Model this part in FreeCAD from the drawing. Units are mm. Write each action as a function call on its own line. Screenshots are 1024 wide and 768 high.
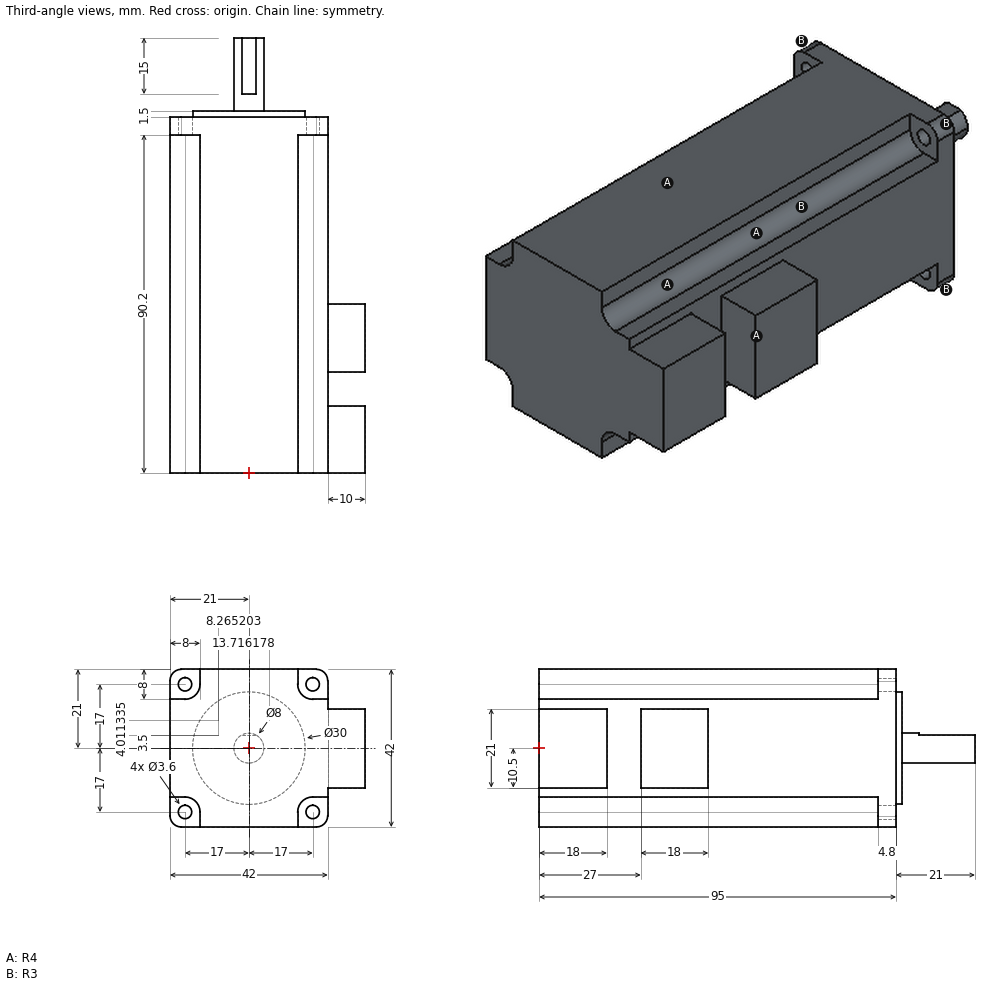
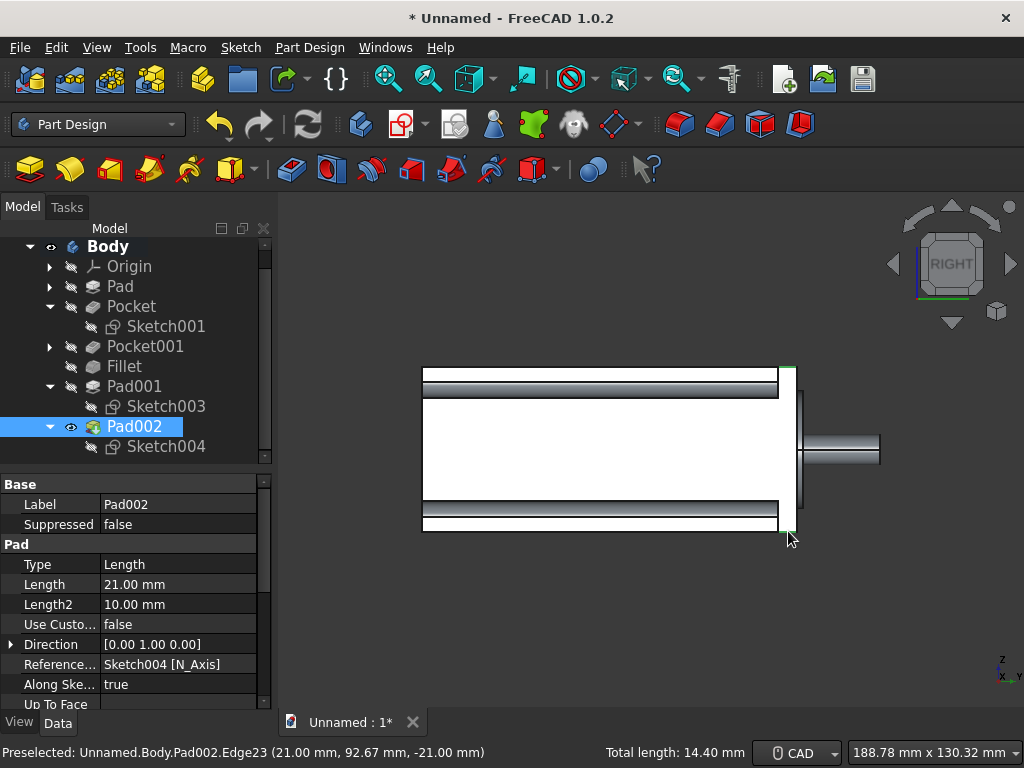
scroll(788, 531, up, 4)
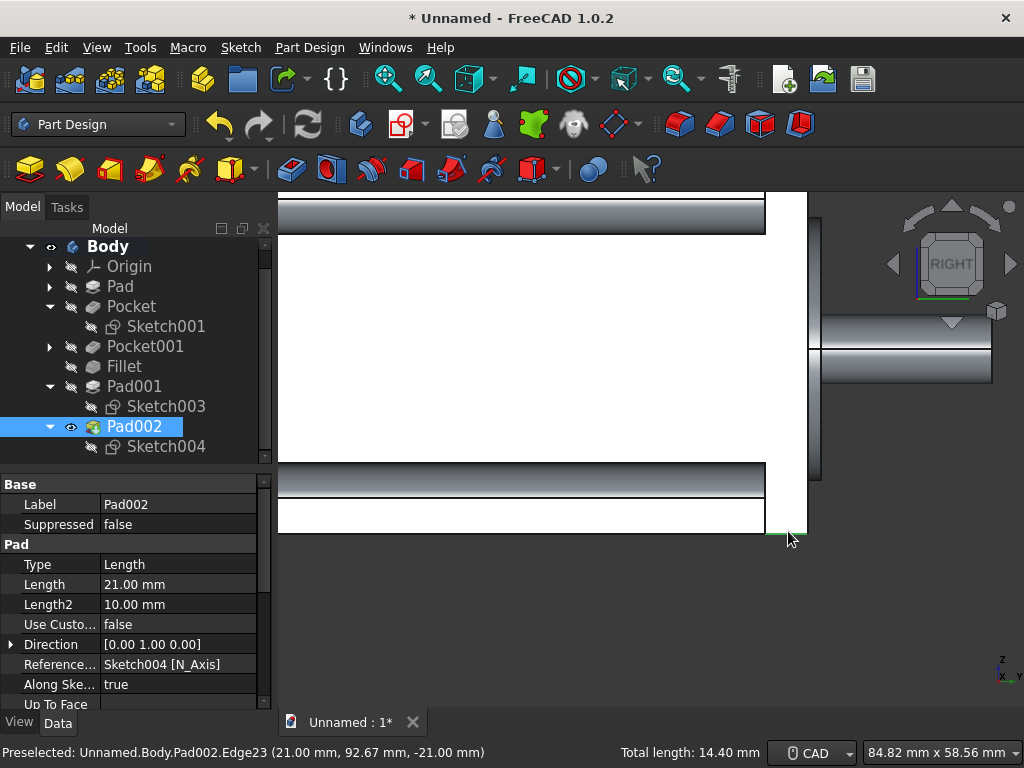
click(390, 80)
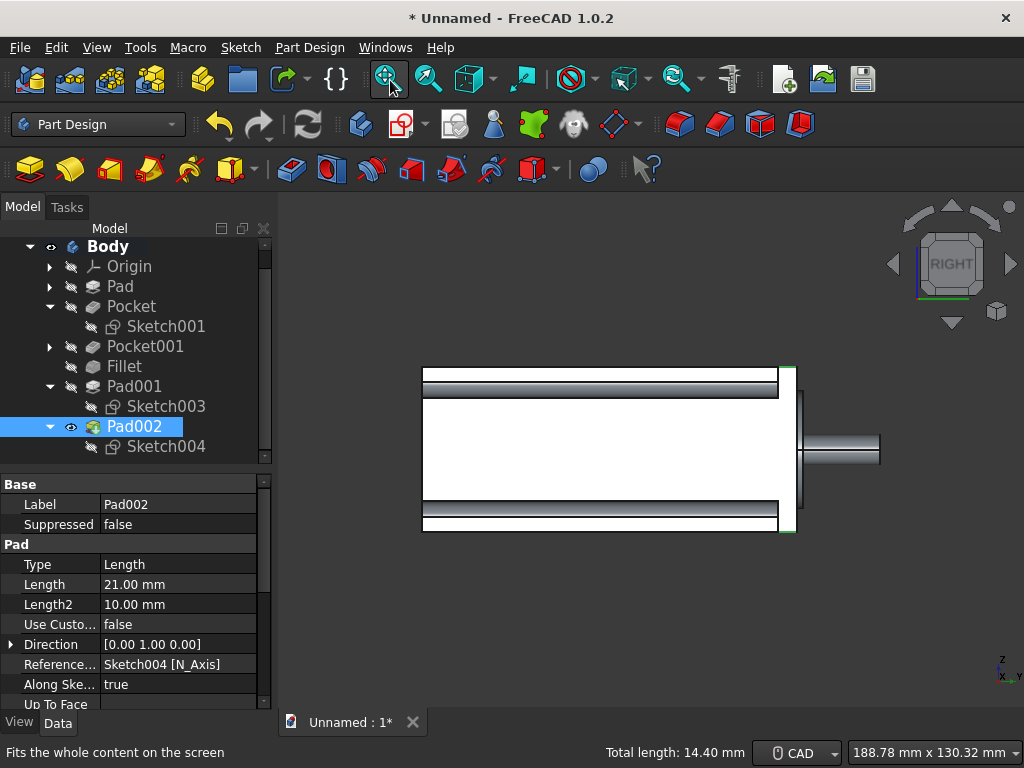
key(5)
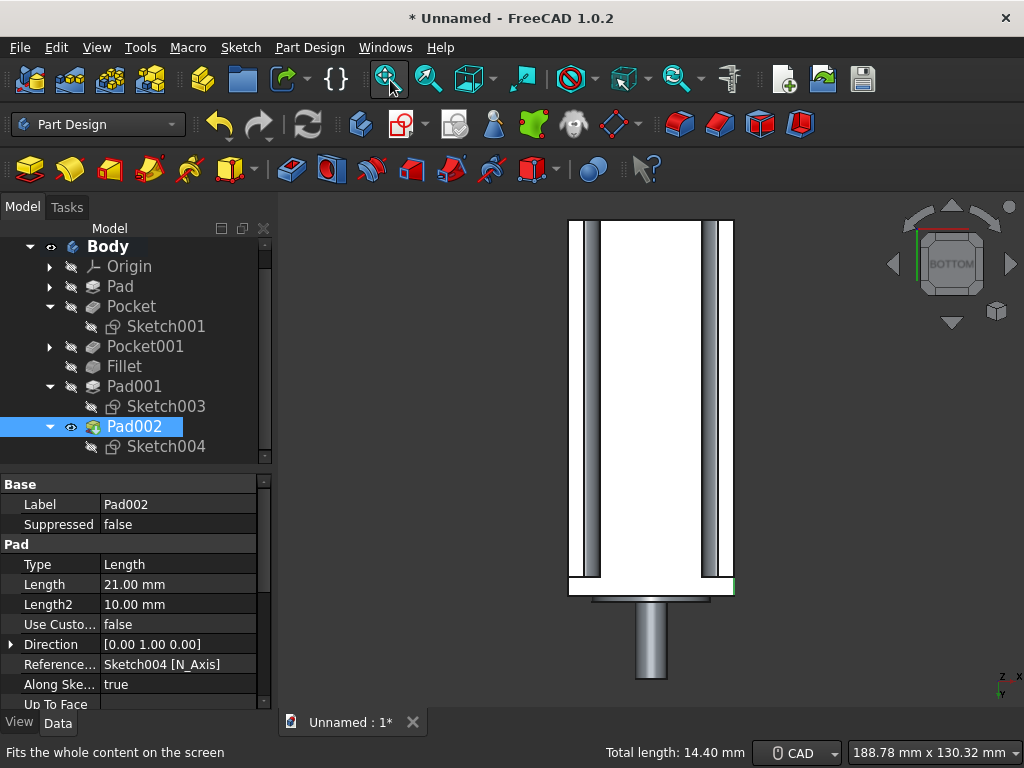
click(568, 585, ctrl)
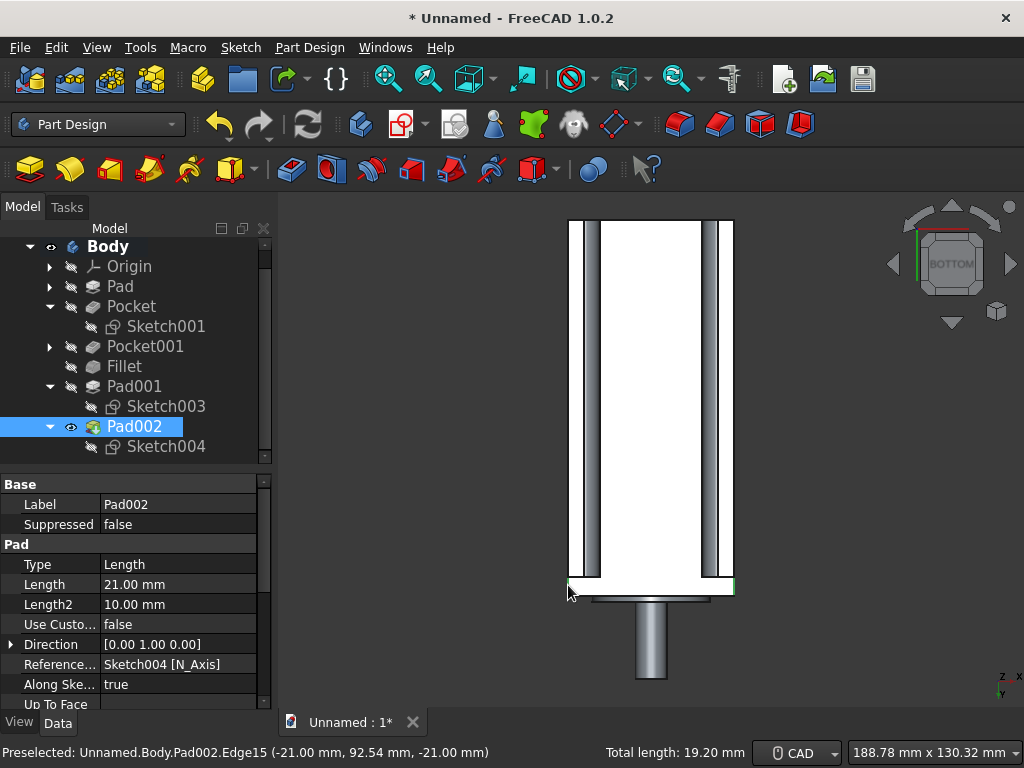
click(680, 124)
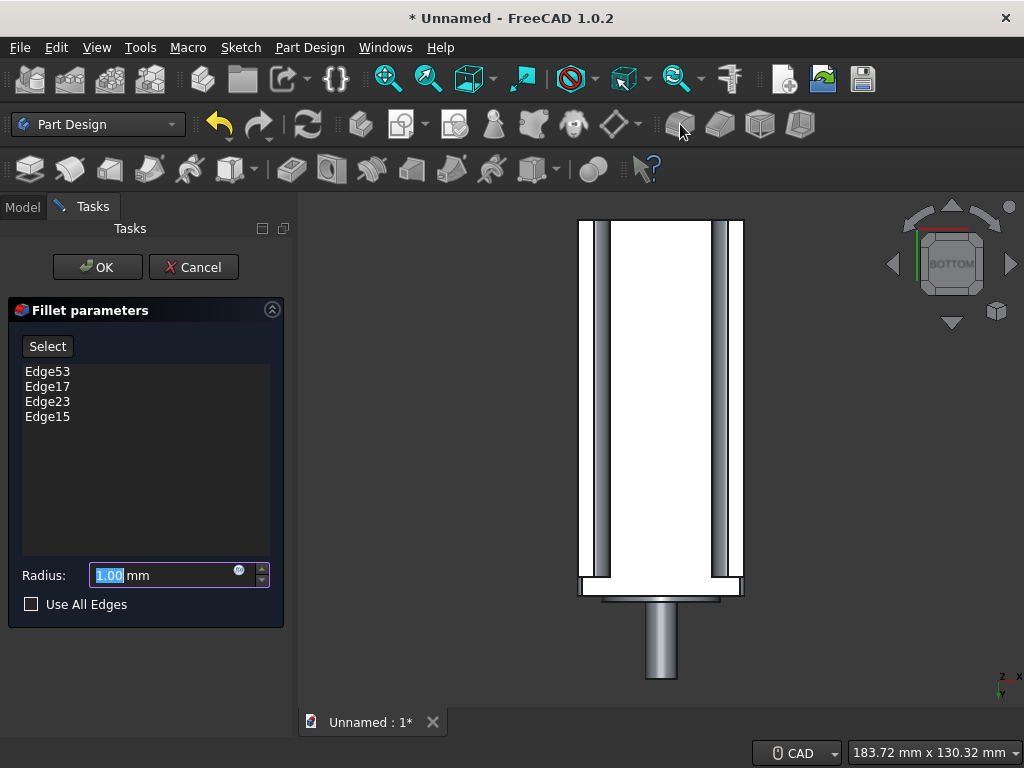
text(3)
key(Tab)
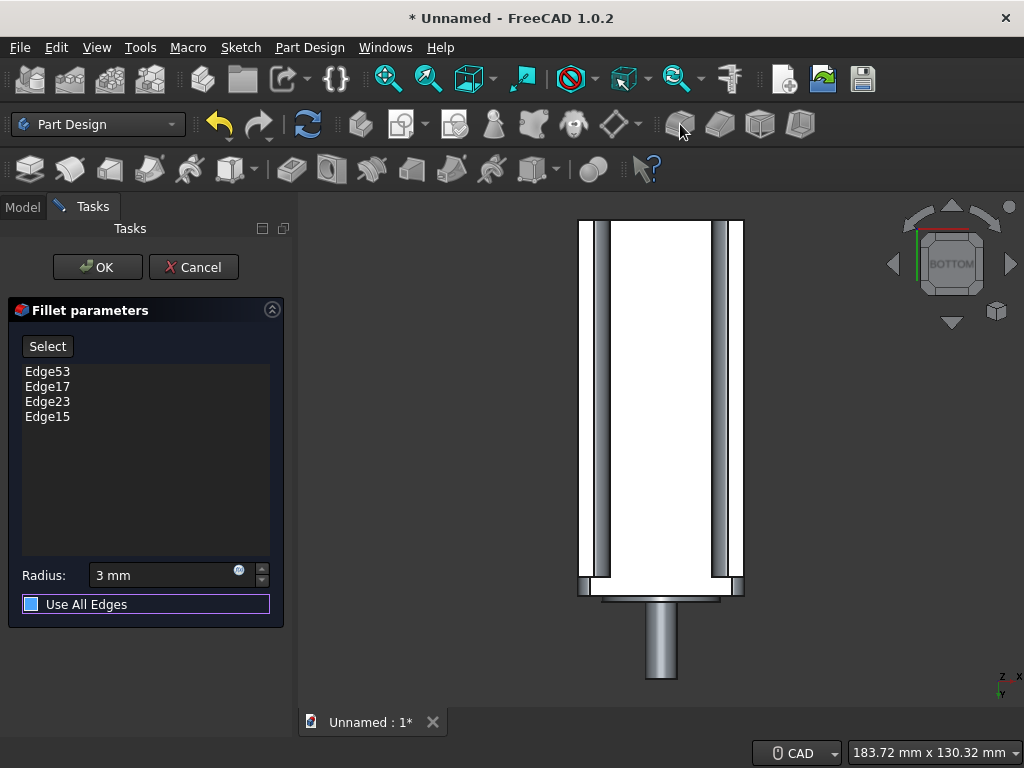
click(98, 267)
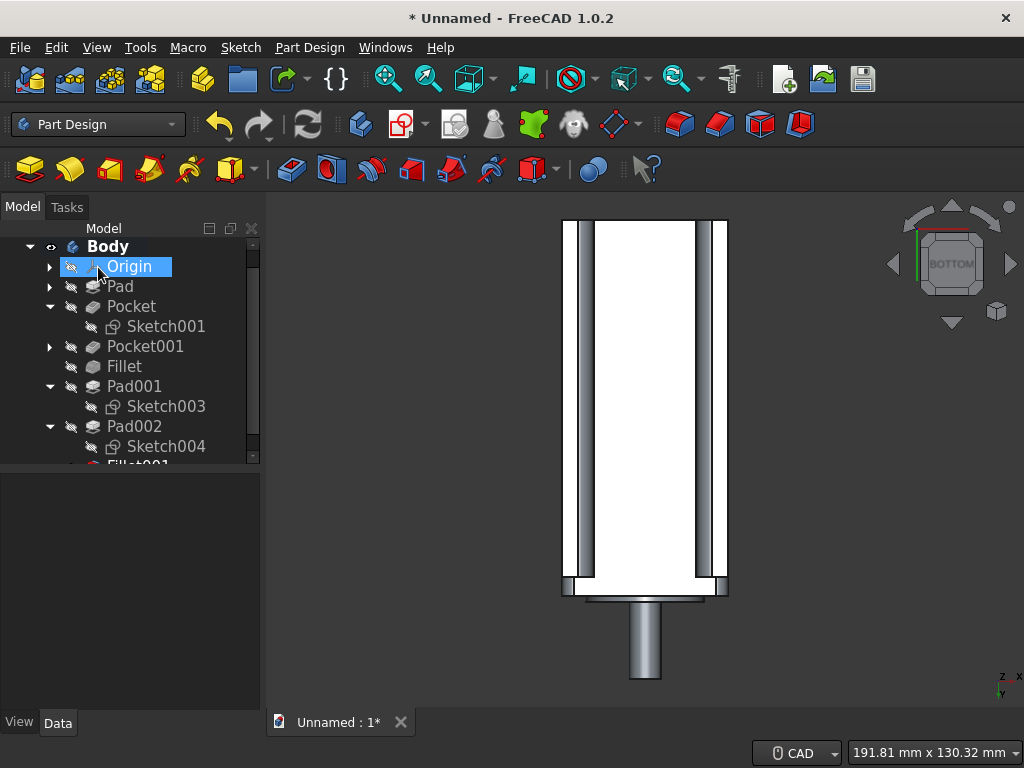
key(0)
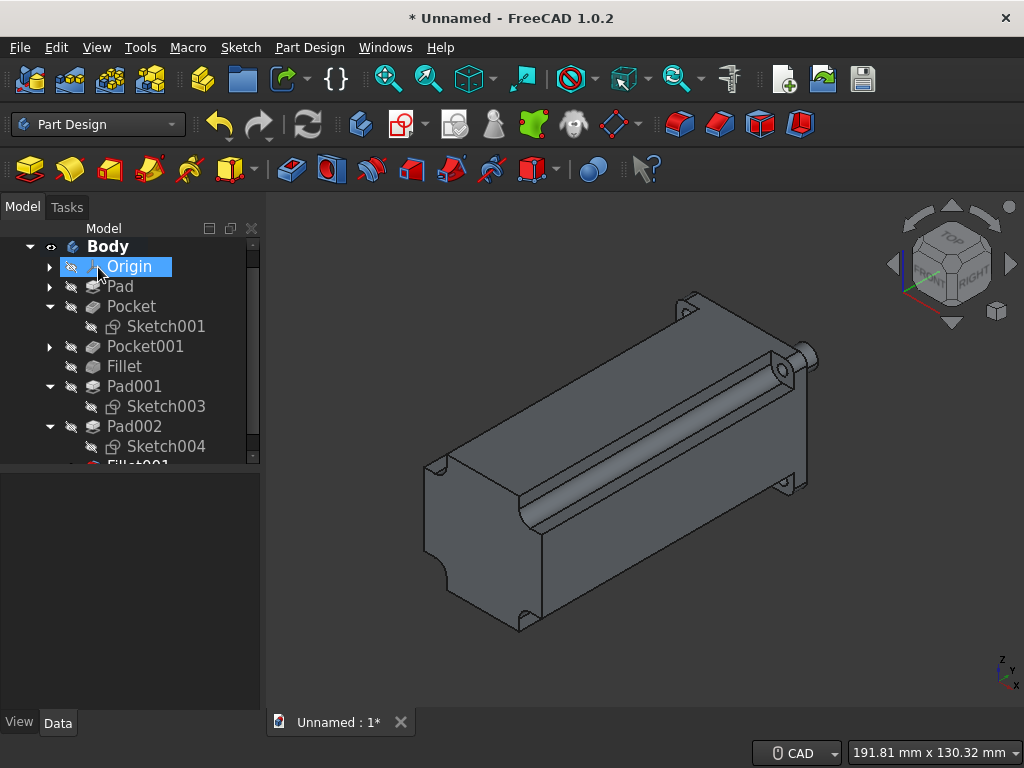
click(750, 456)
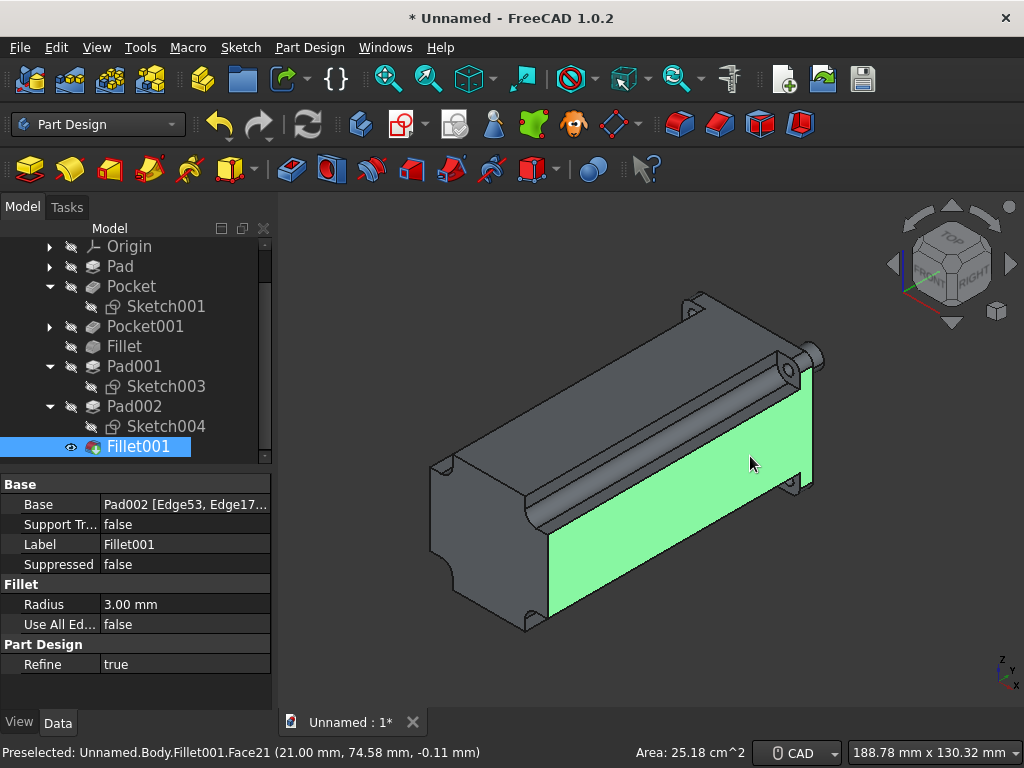
click(402, 124)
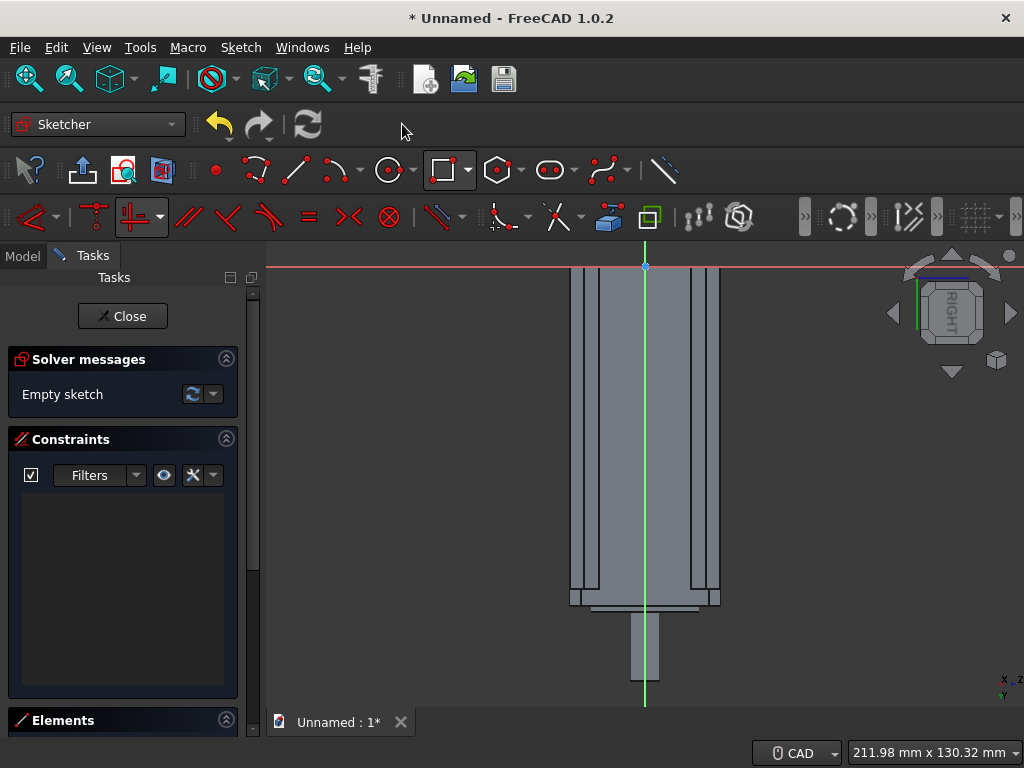
scroll(576, 474, down, 5)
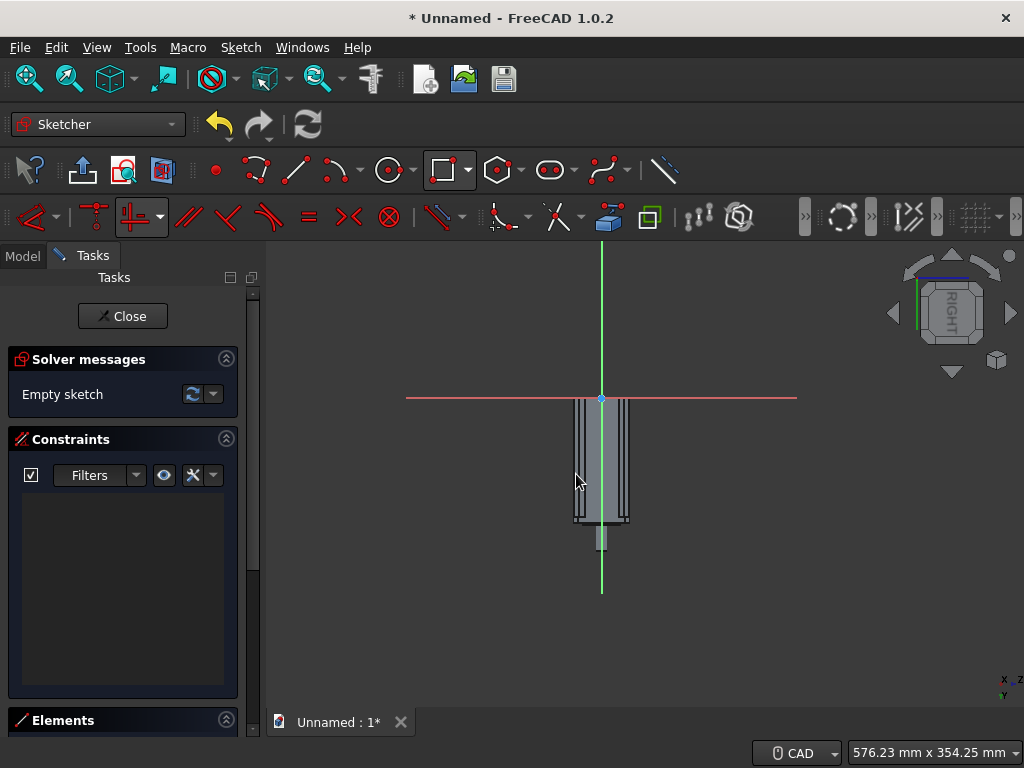
scroll(608, 416, up, 8)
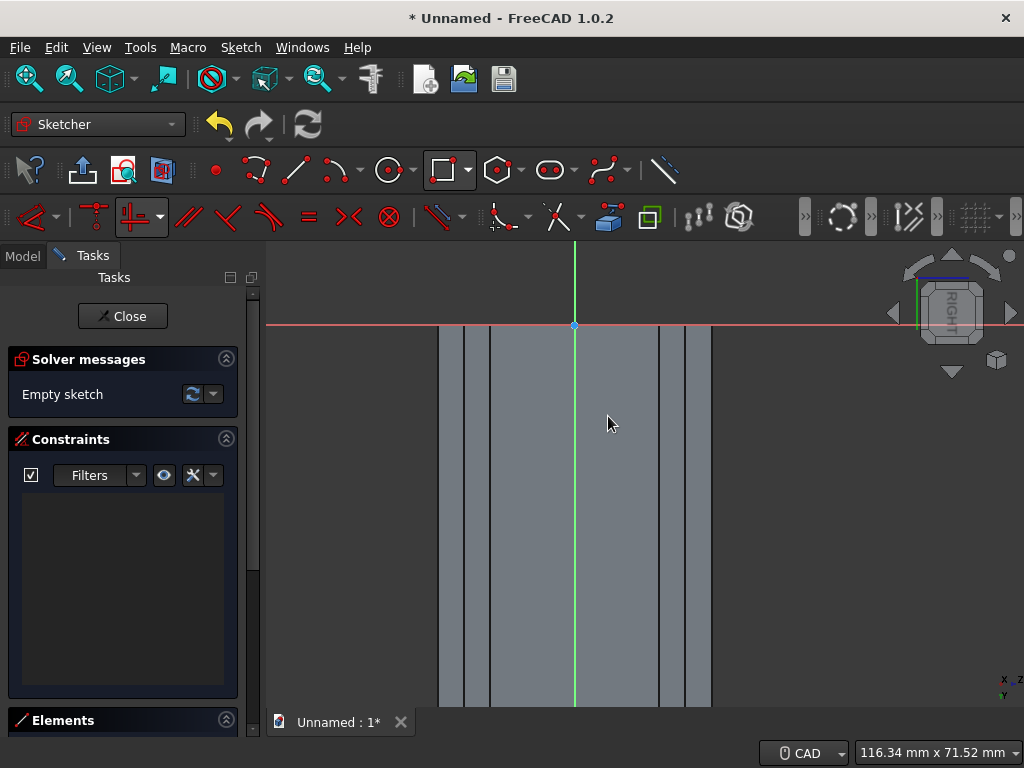
click(444, 170)